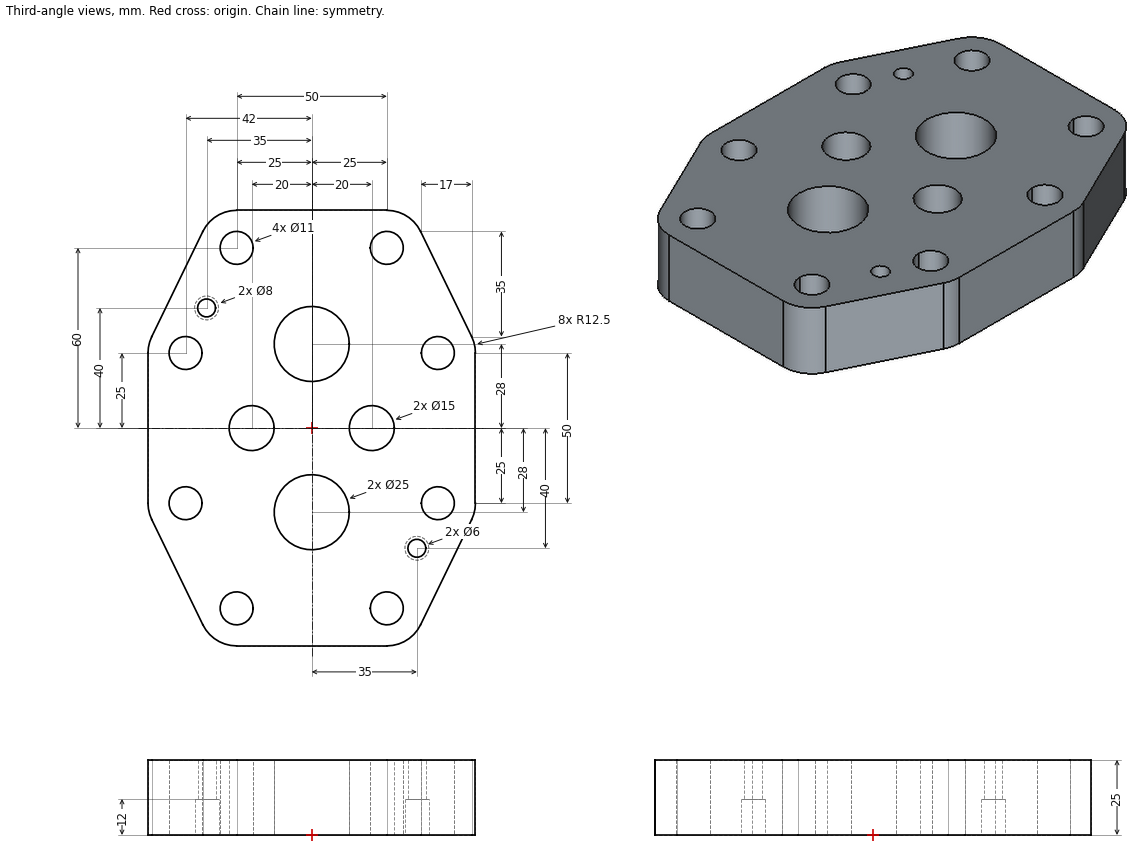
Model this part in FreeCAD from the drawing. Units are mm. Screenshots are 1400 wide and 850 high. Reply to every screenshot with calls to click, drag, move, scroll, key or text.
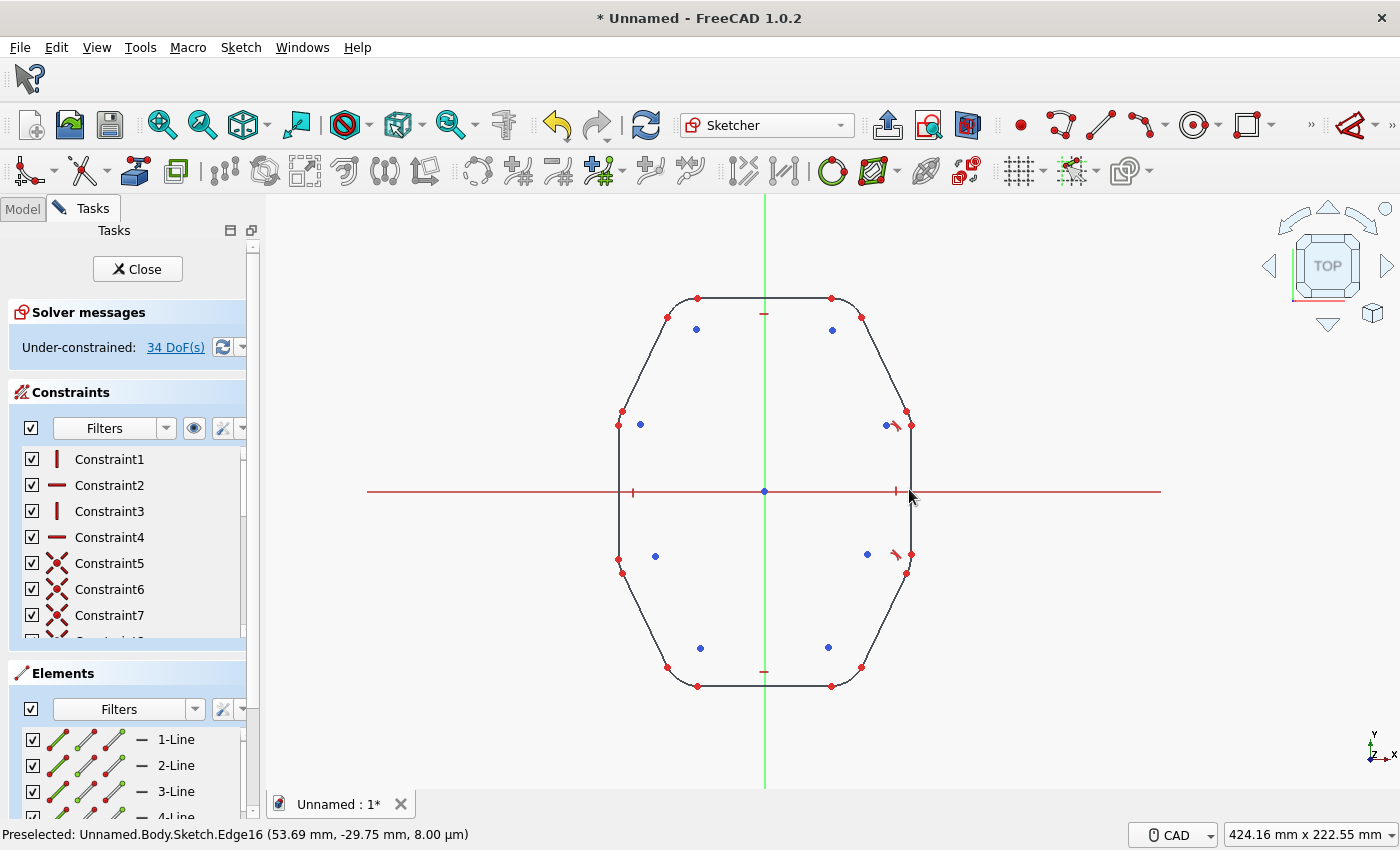
click(893, 383)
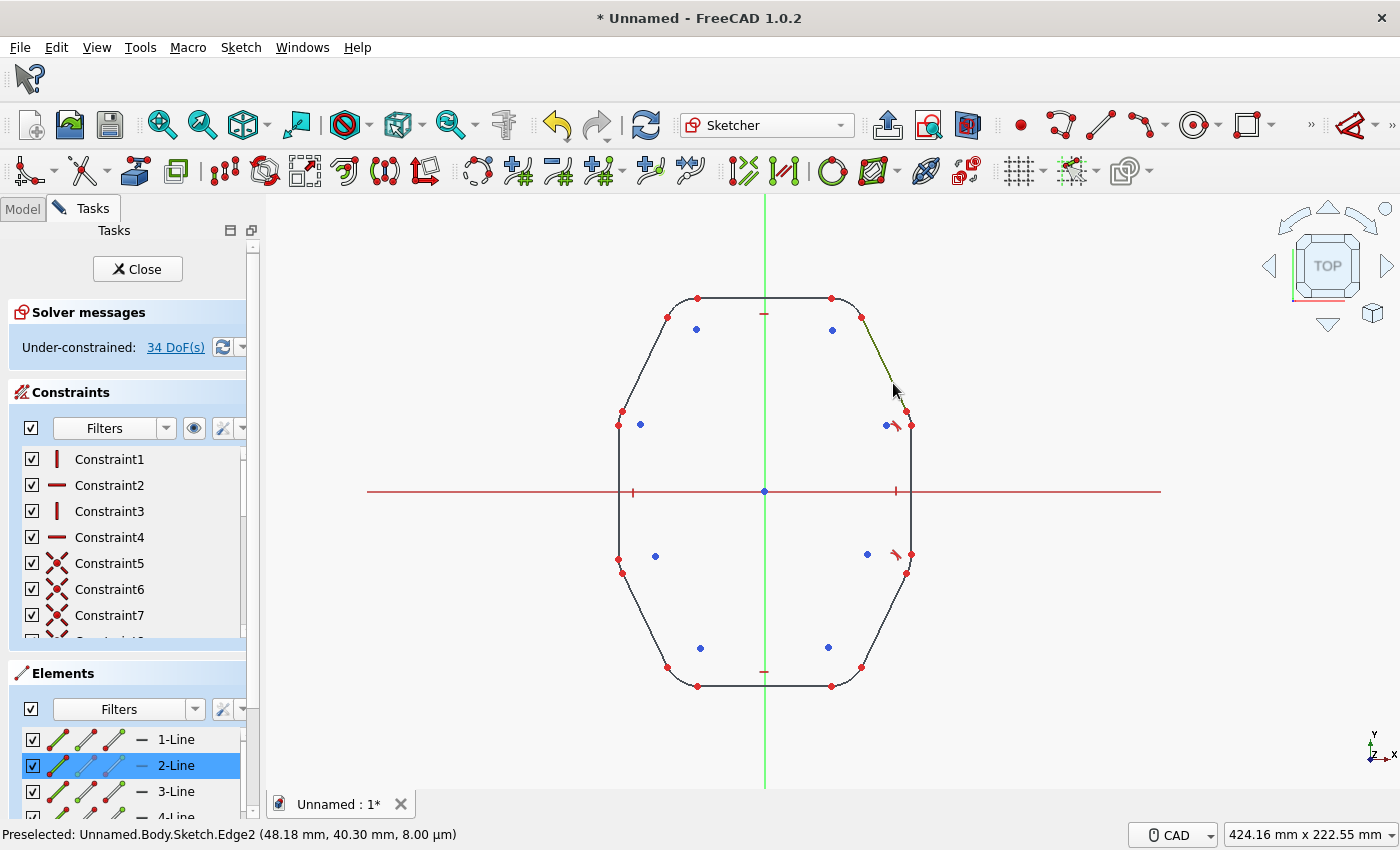
scroll(910, 418, up, 4)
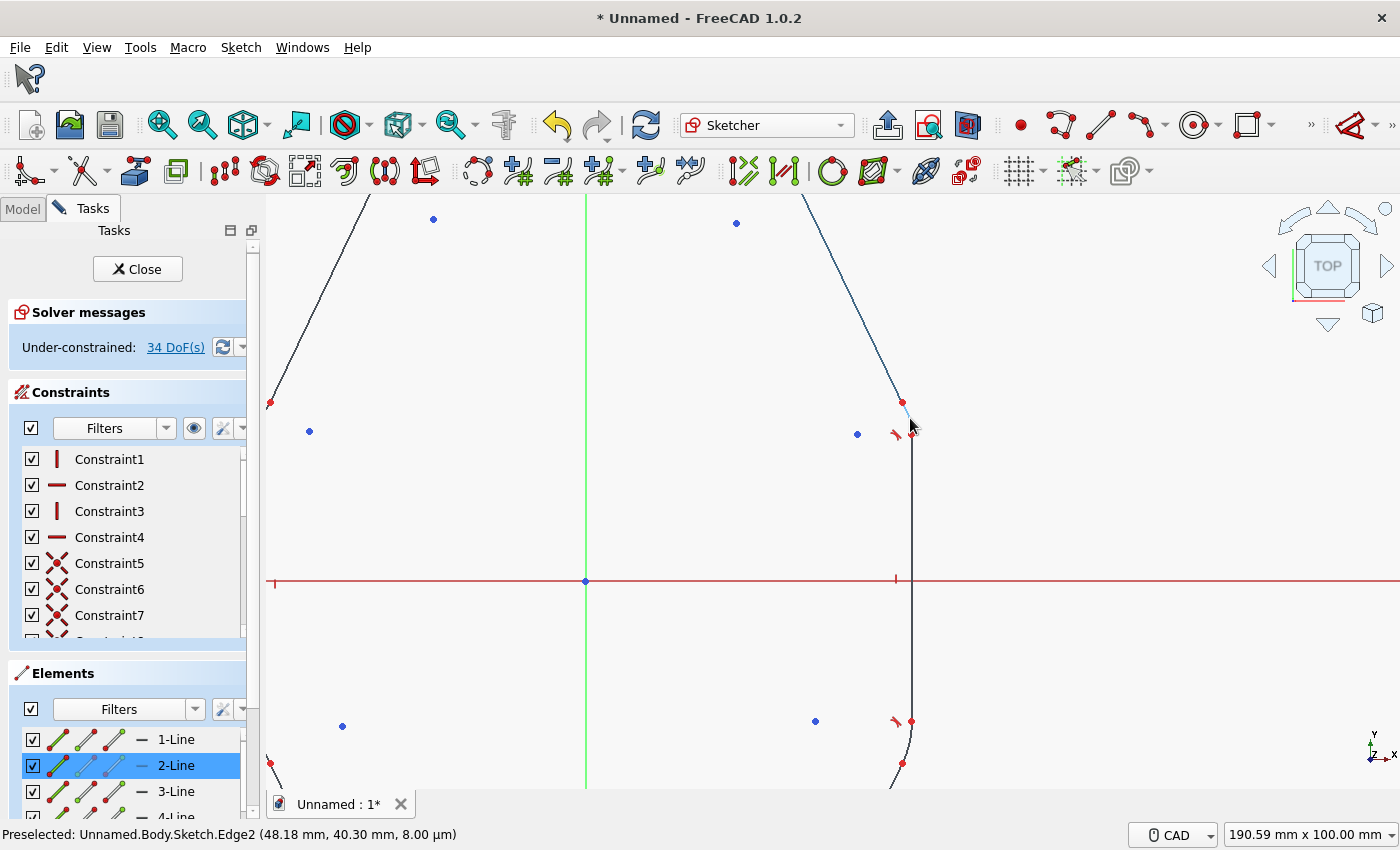
click(909, 418)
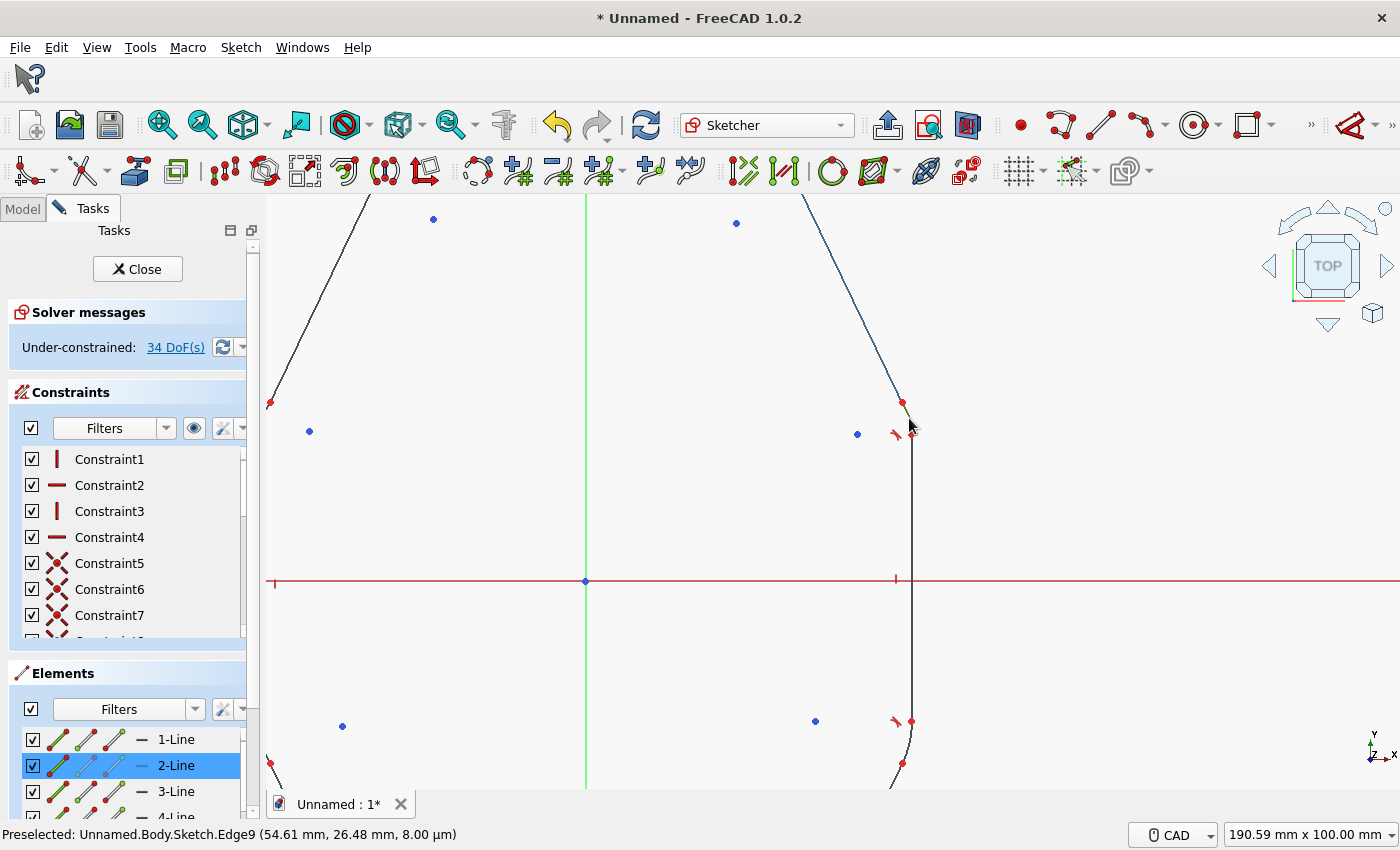
key(t)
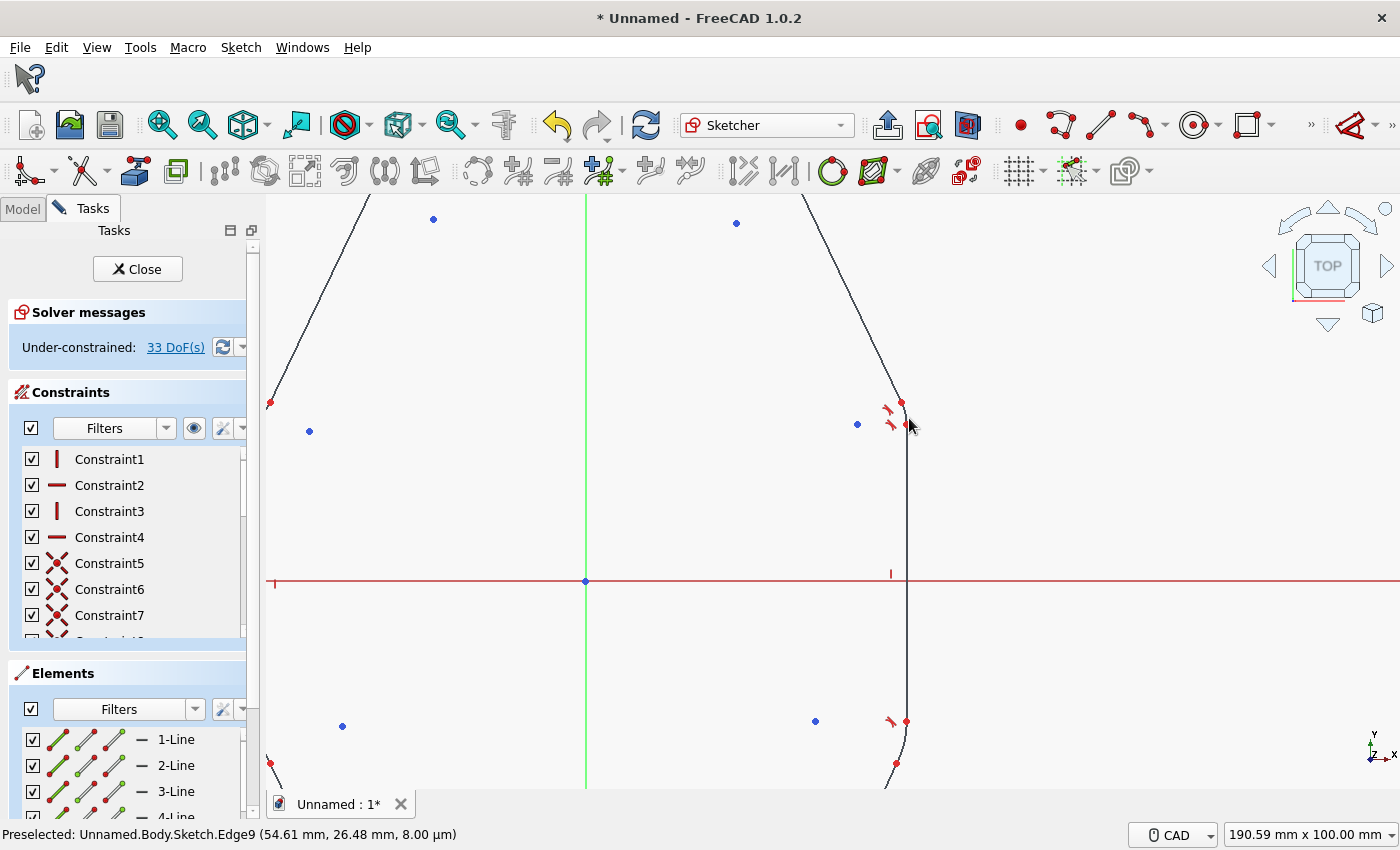
click(872, 340)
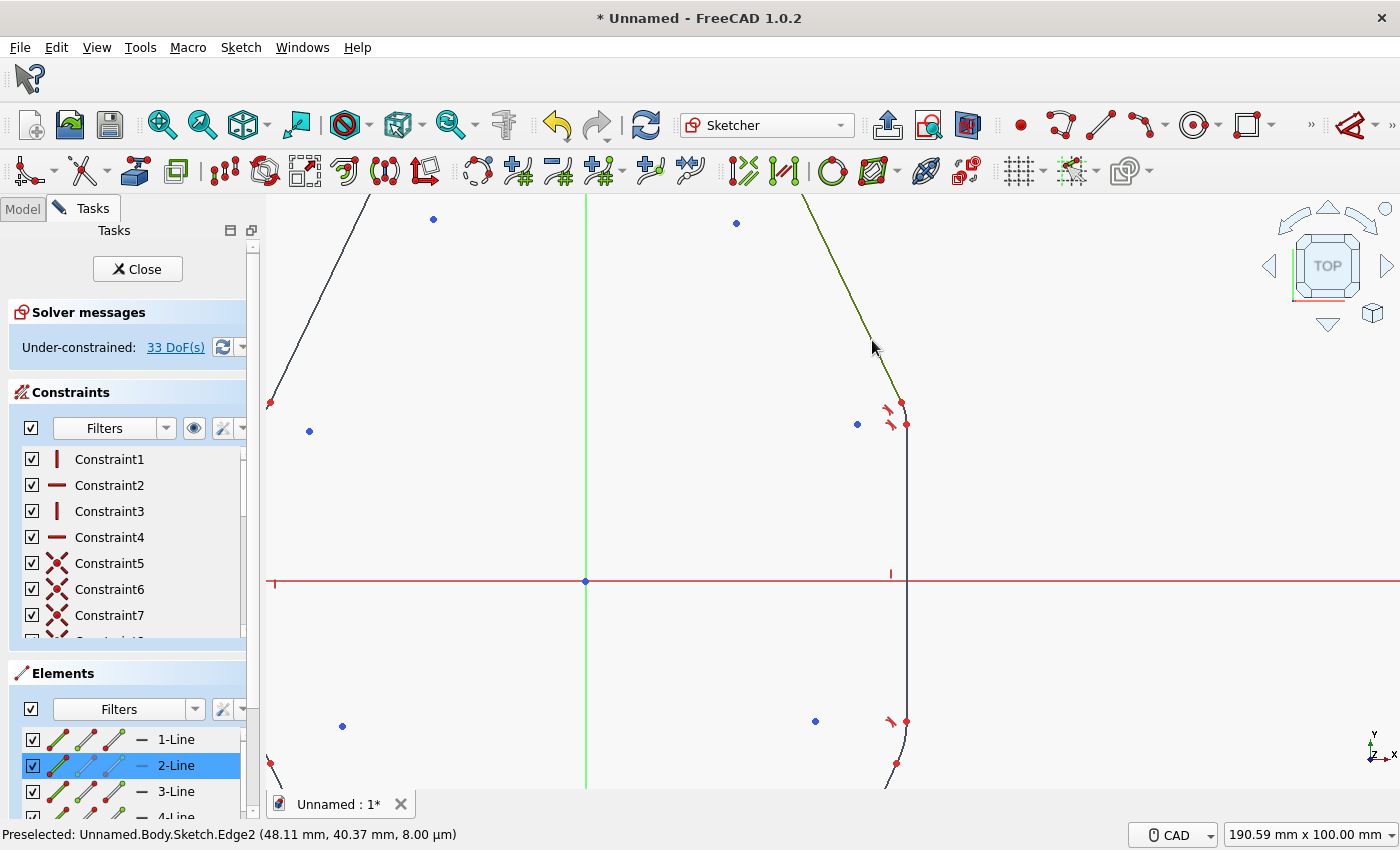
scroll(910, 418, down, 4)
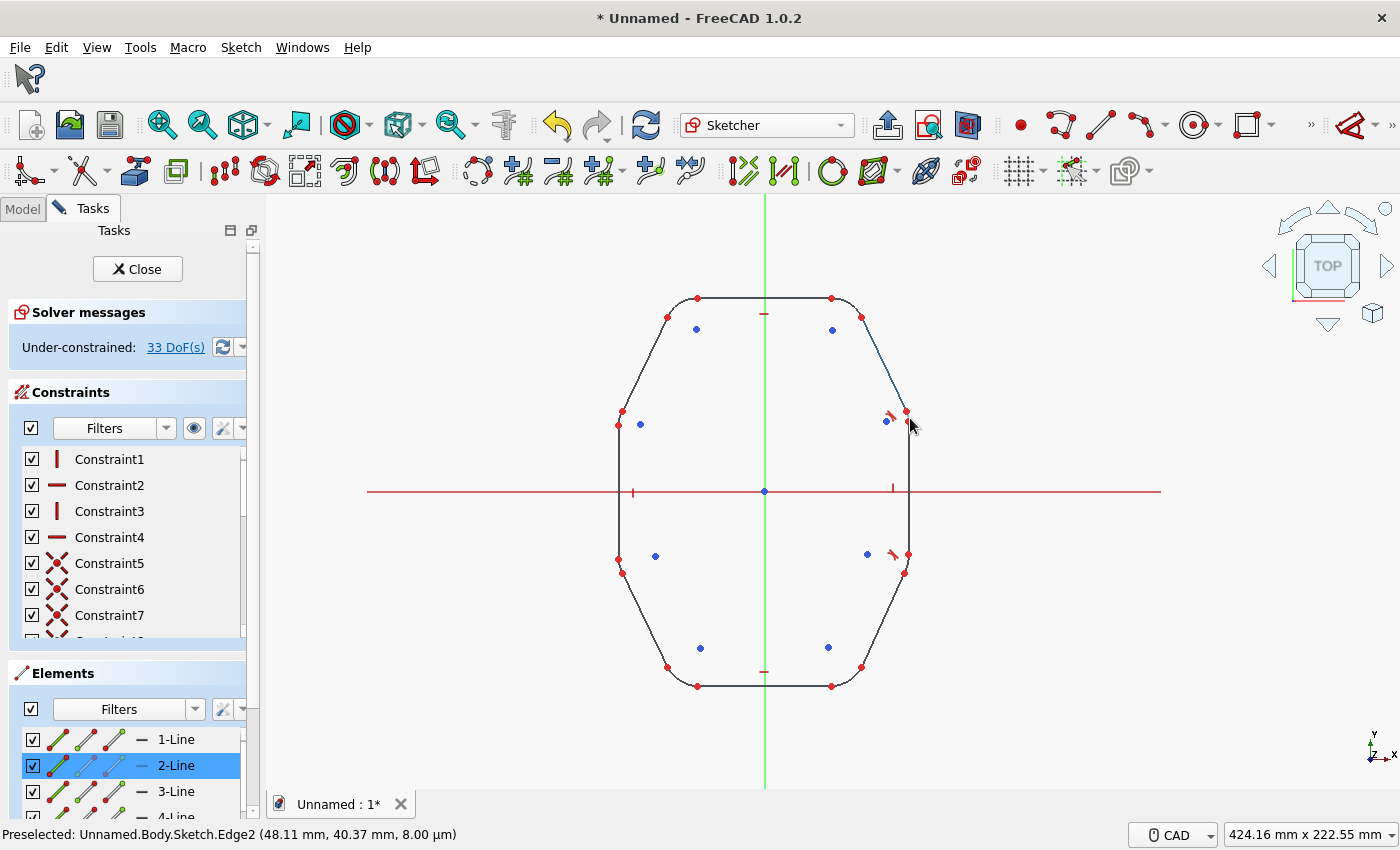
scroll(855, 308, up, 2)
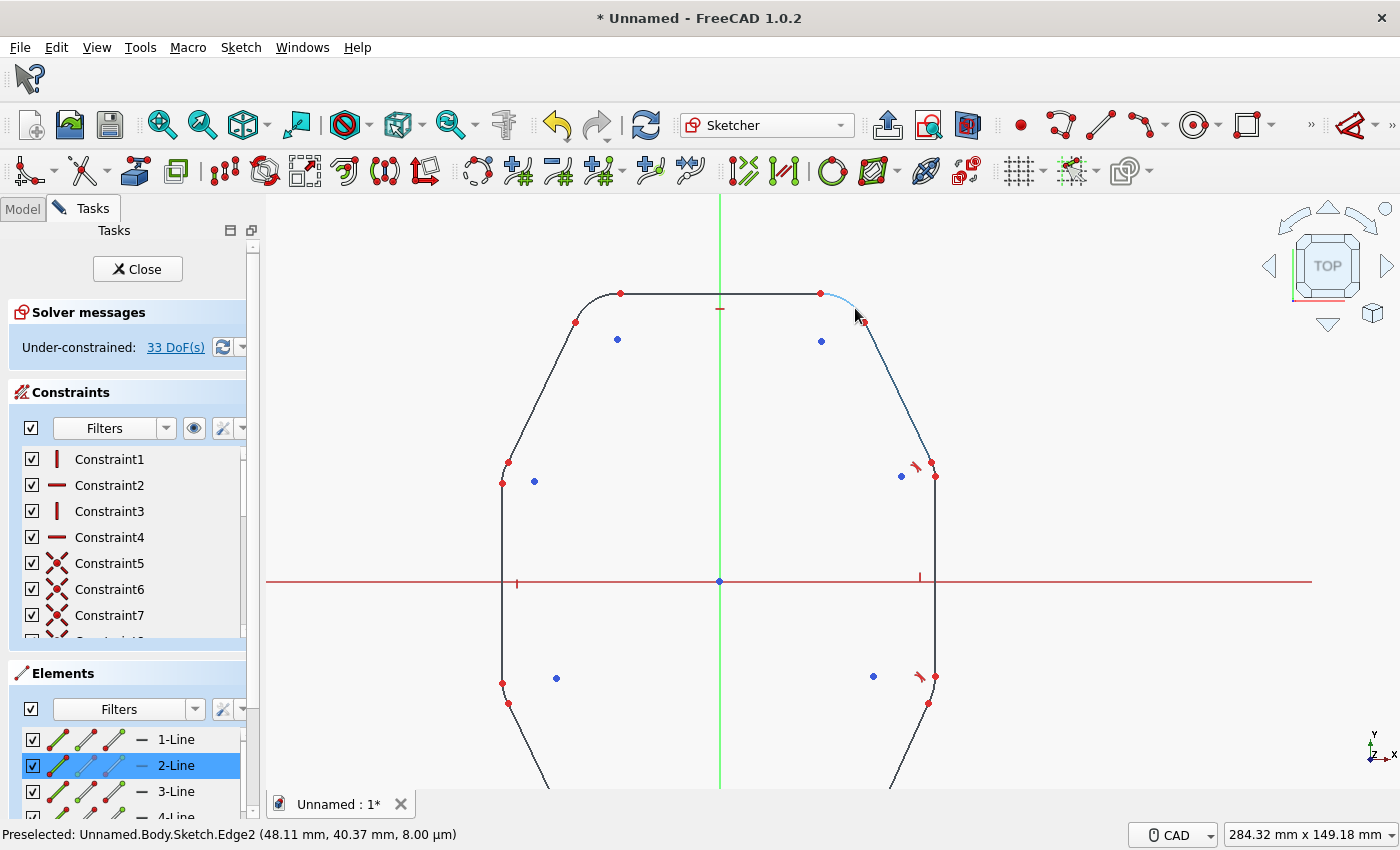
click(855, 308)